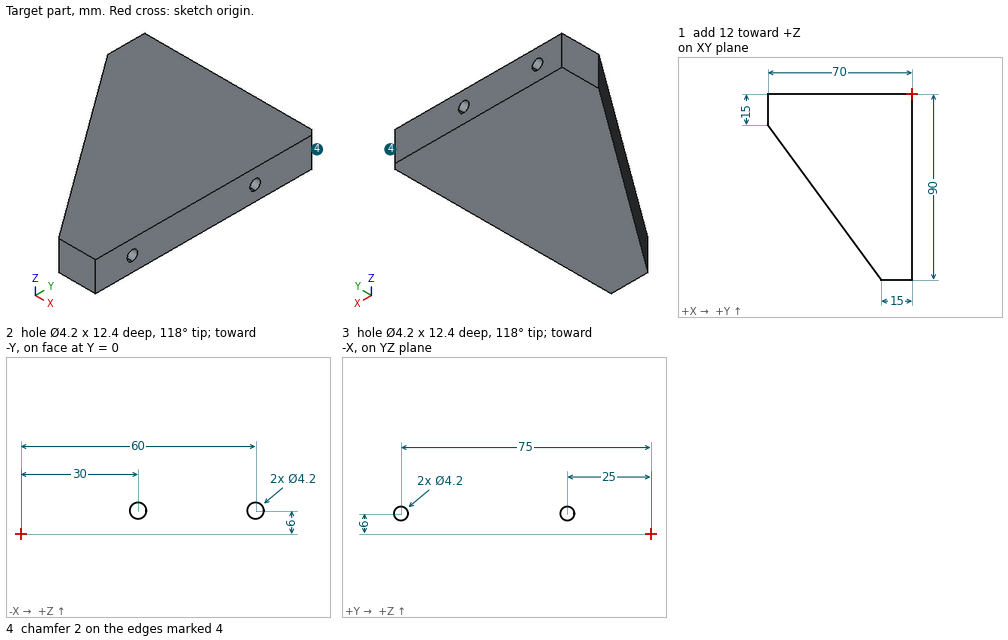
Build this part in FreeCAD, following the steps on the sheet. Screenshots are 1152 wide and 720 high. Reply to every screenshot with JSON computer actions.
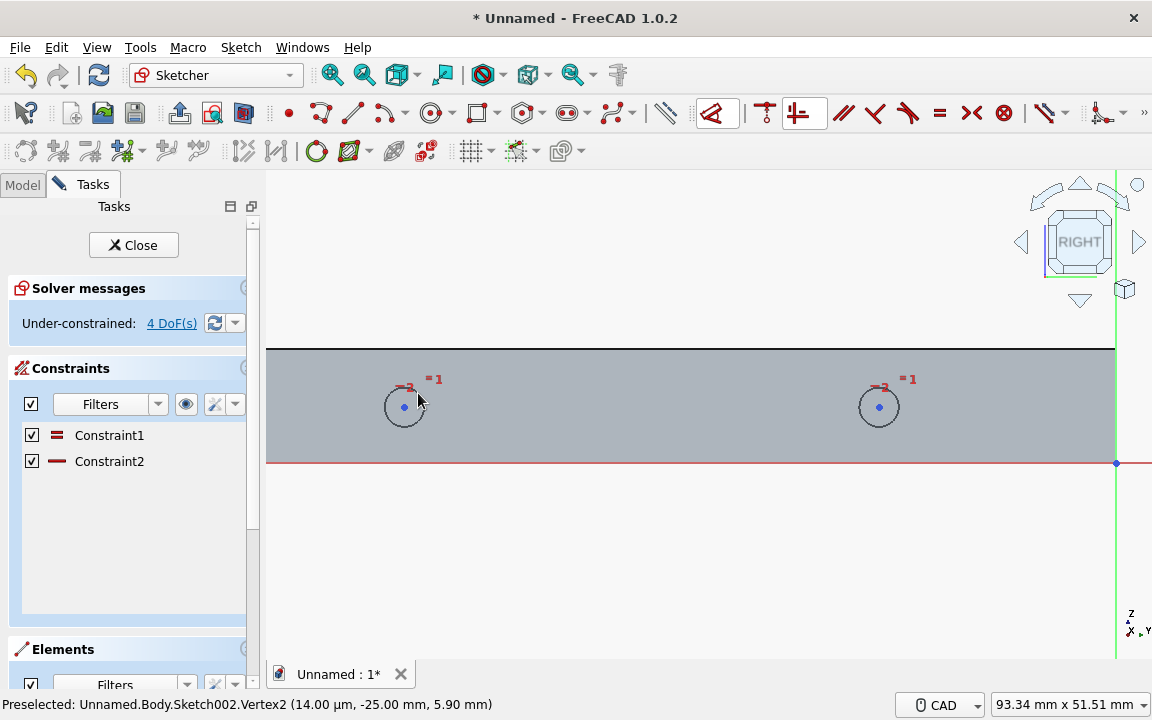
{"action": "left_click", "coordinate": [418, 393]}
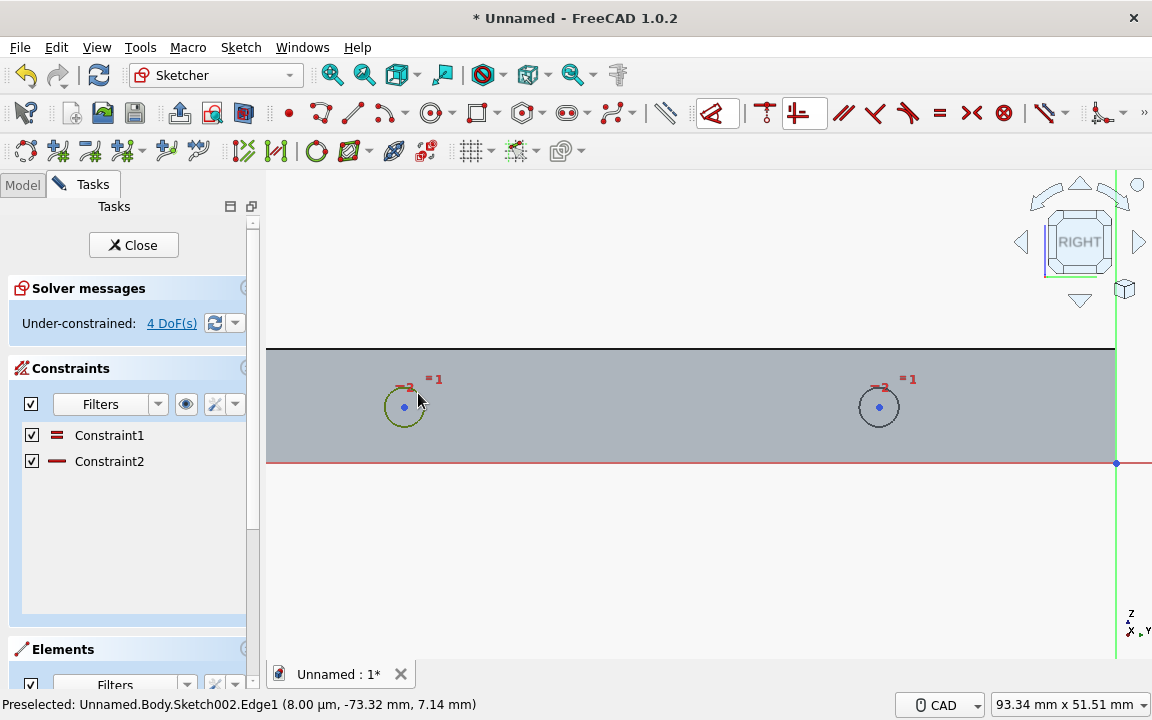
{"action": "key", "text": "k o"}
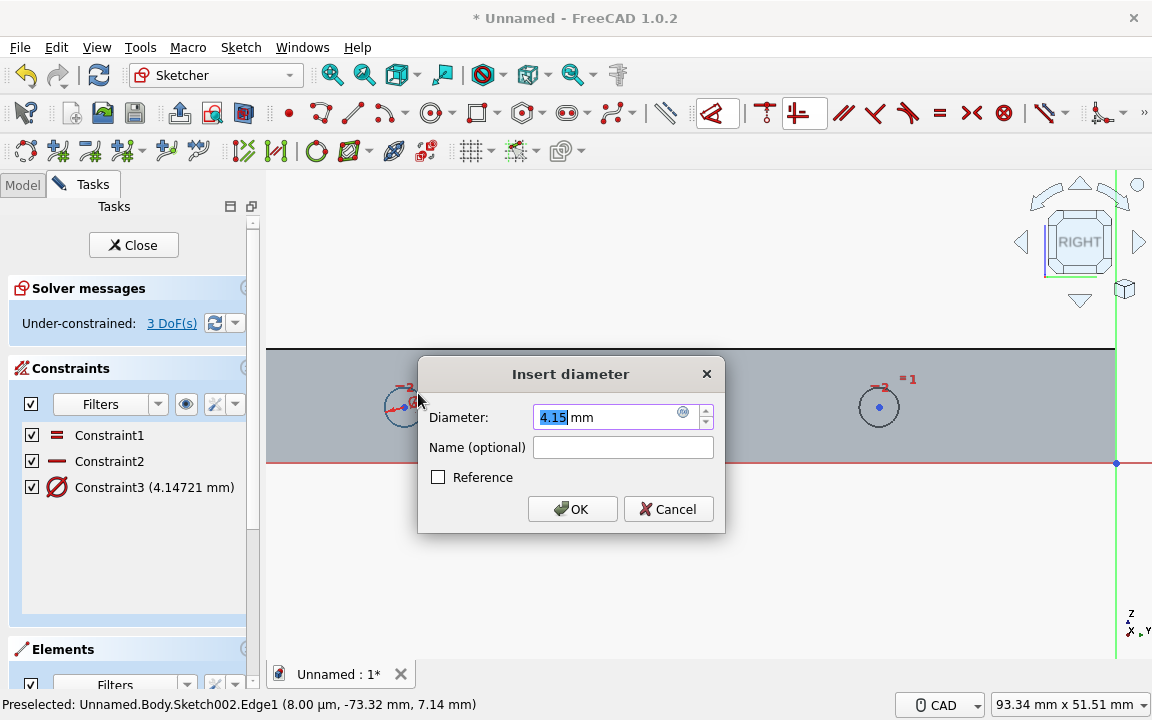
{"action": "type", "text": "4.2"}
{"action": "key", "text": "Return"}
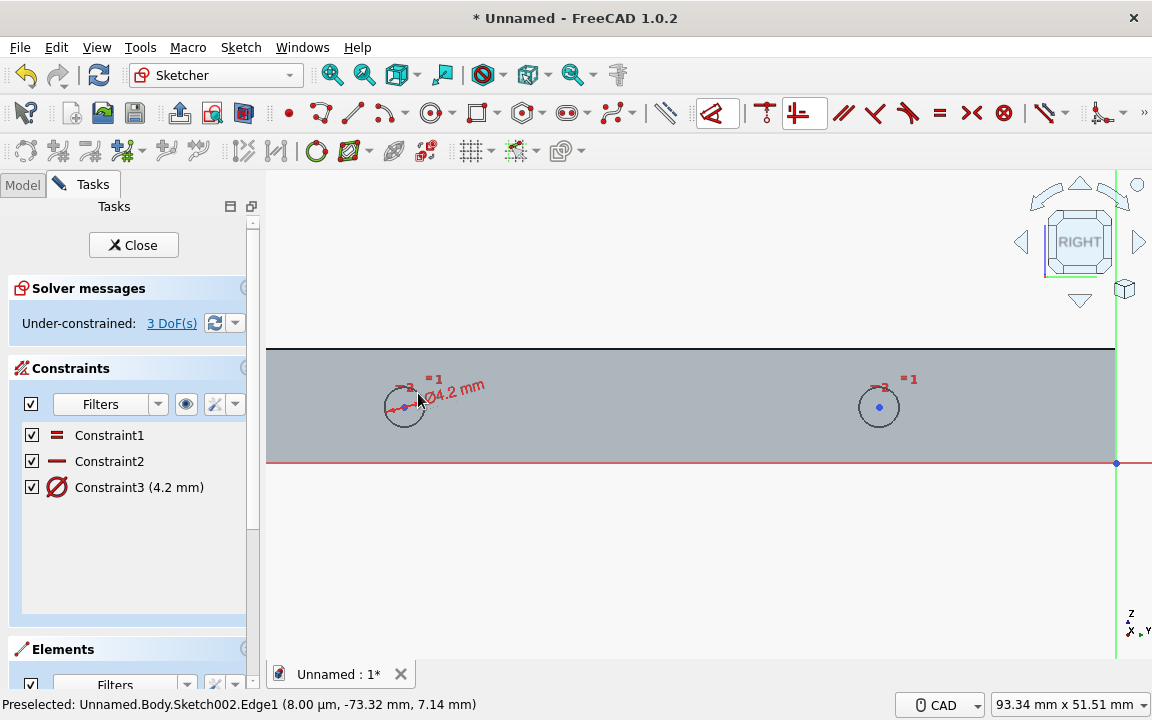
{"action": "left_click", "coordinate": [404, 407]}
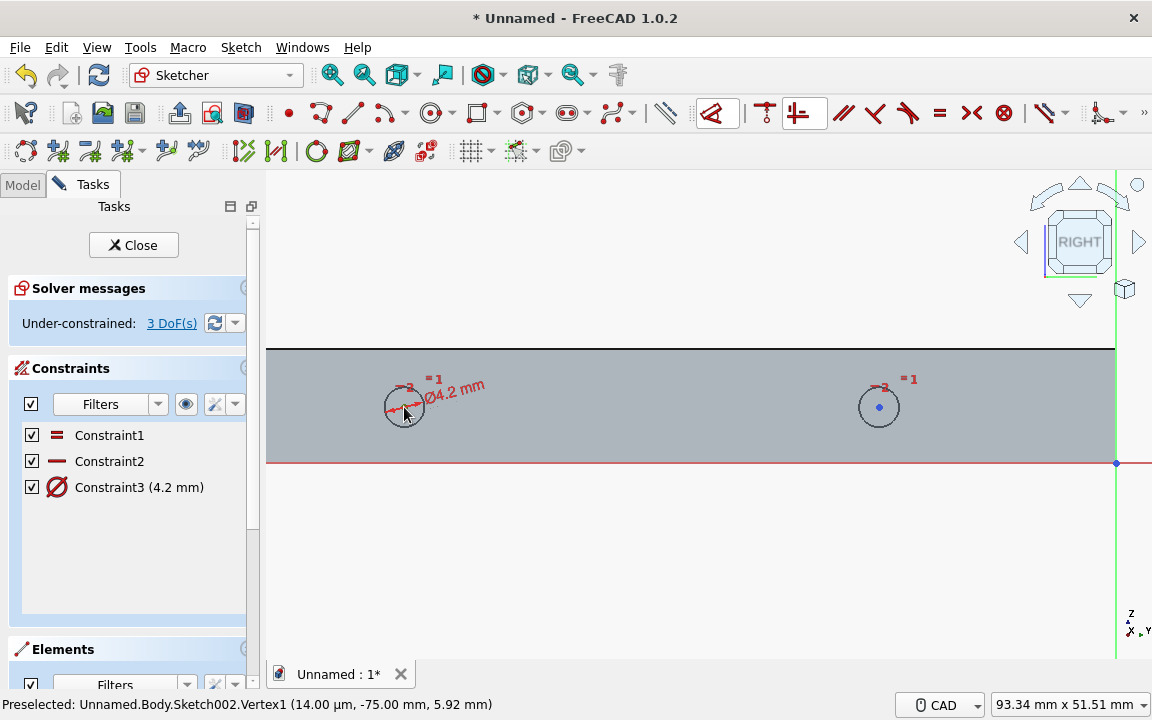
{"action": "key", "text": "i"}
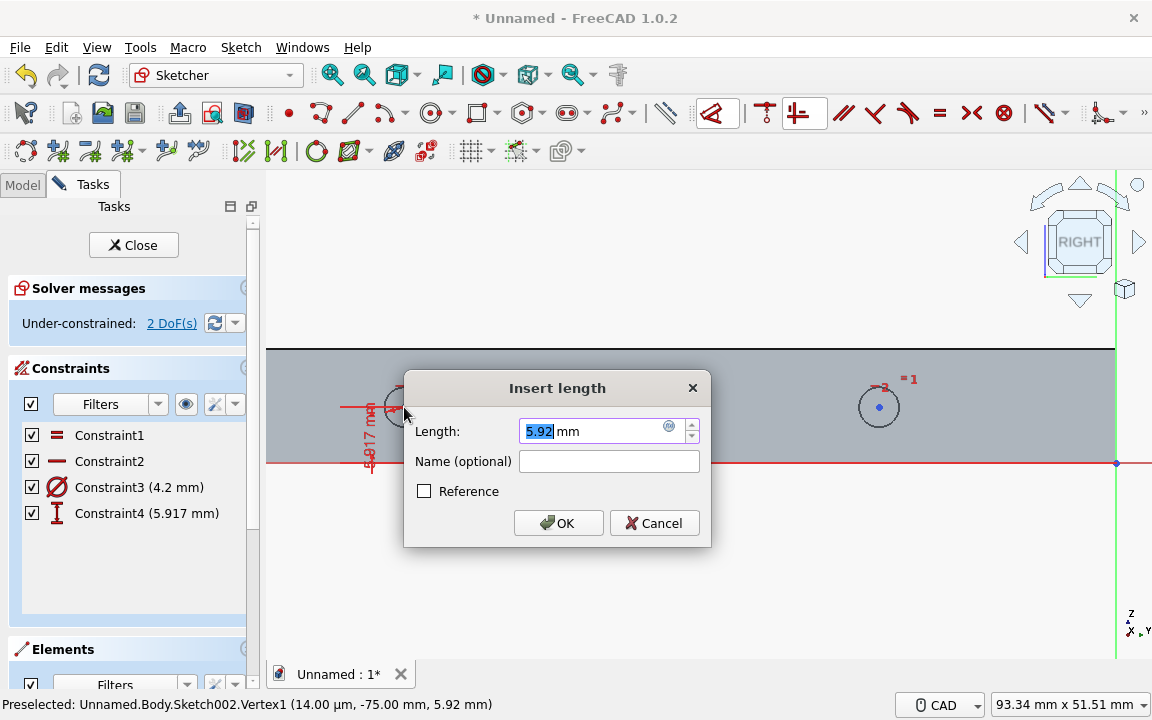
{"action": "type", "text": "6"}
{"action": "key", "text": "Return"}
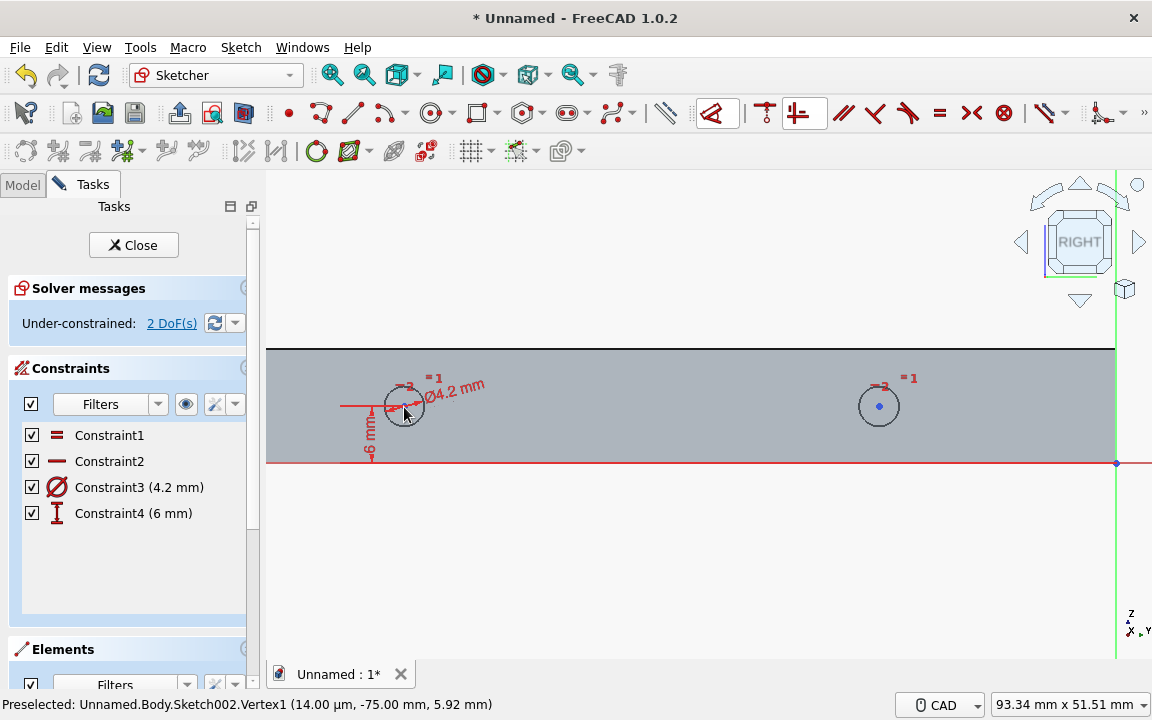
{"action": "left_click", "coordinate": [404, 406]}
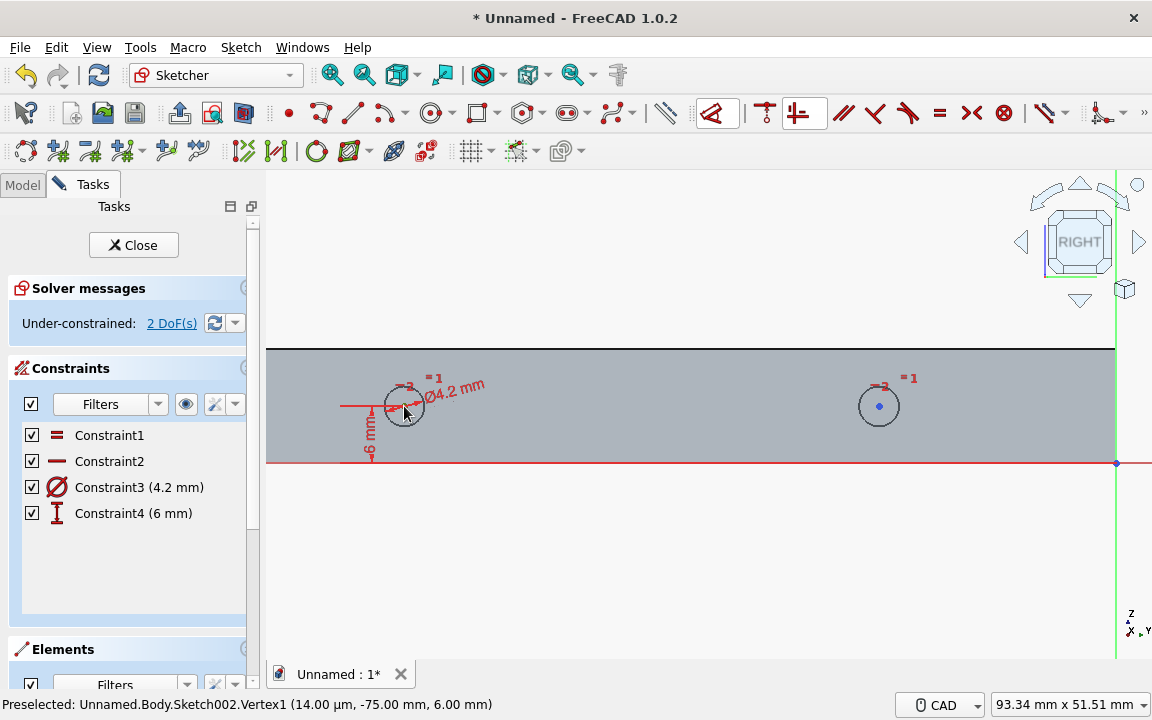
{"action": "left_click", "coordinate": [734, 114]}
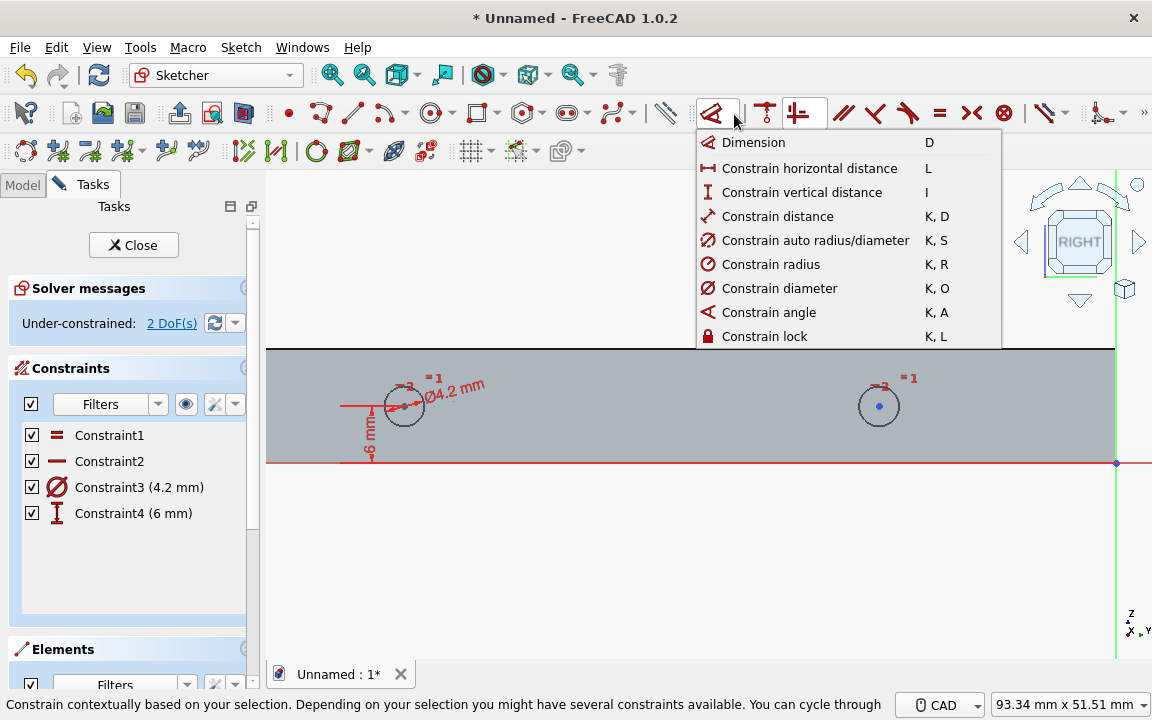
{"action": "left_click", "coordinate": [849, 168]}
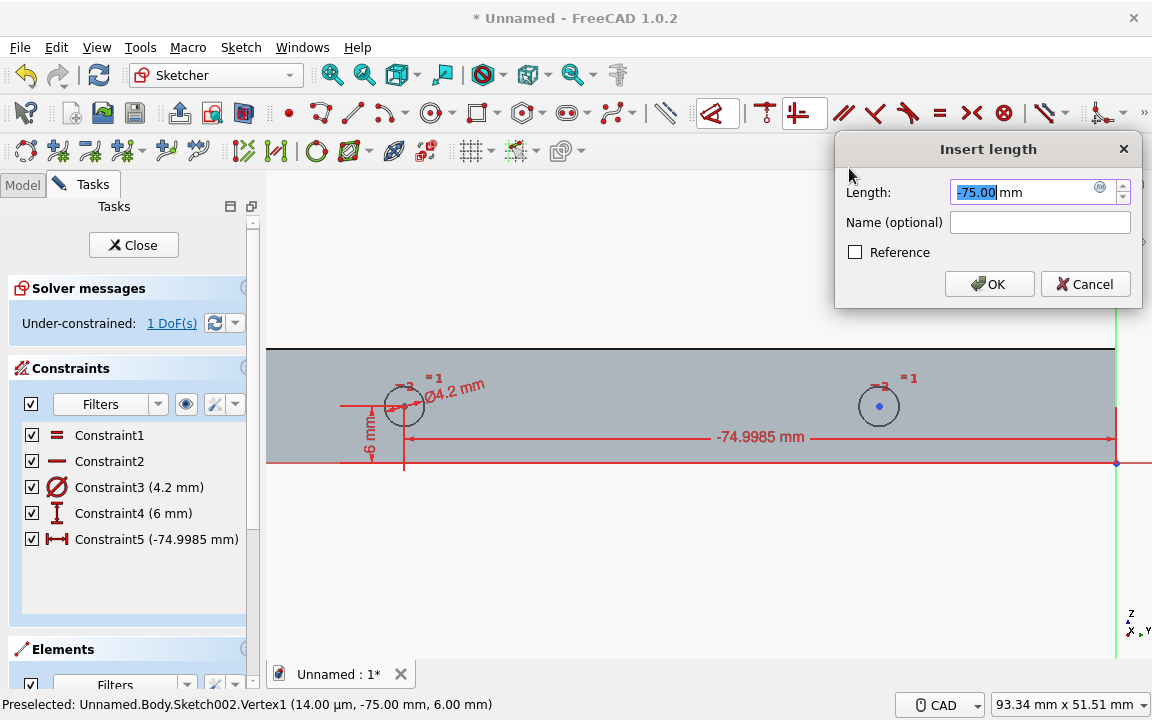
{"action": "type", "text": "-75"}
{"action": "key", "text": "Return"}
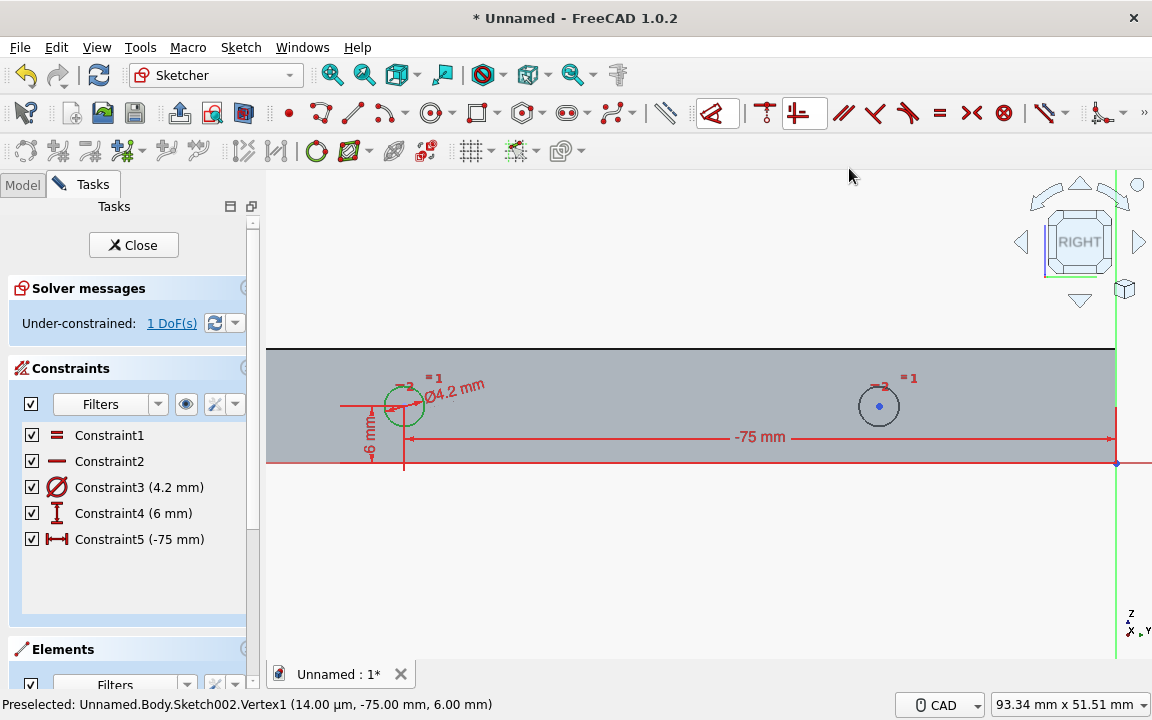
{"action": "left_click", "coordinate": [879, 406]}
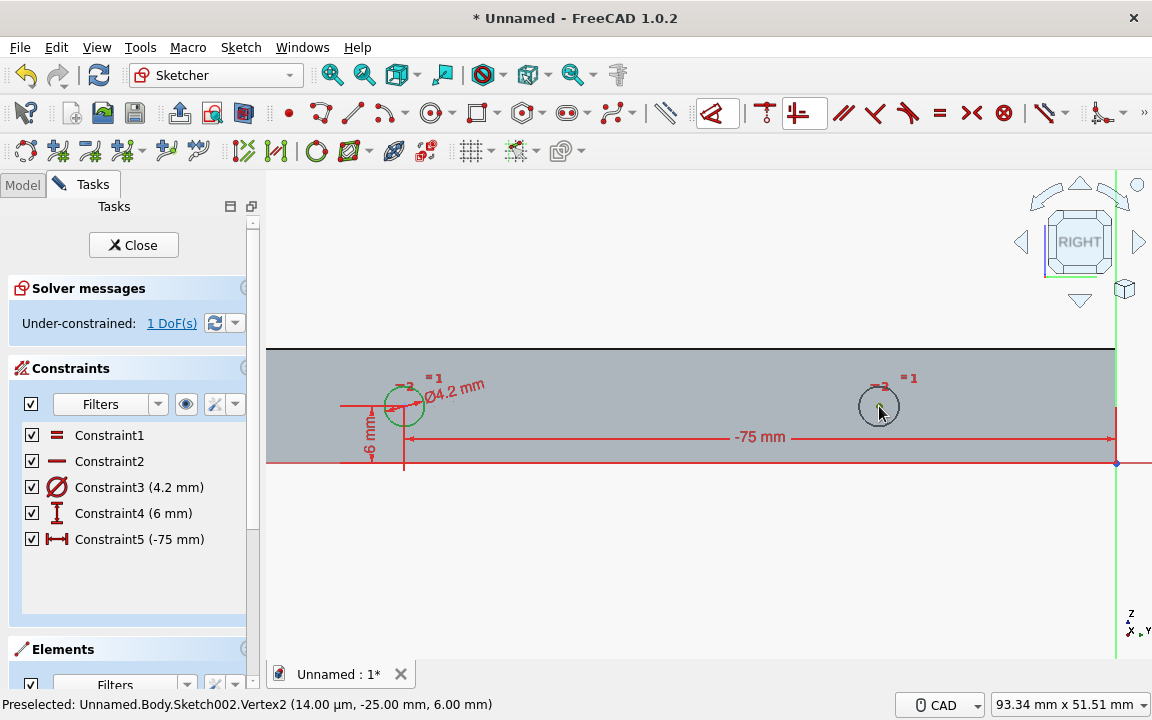
{"action": "left_click", "coordinate": [734, 114]}